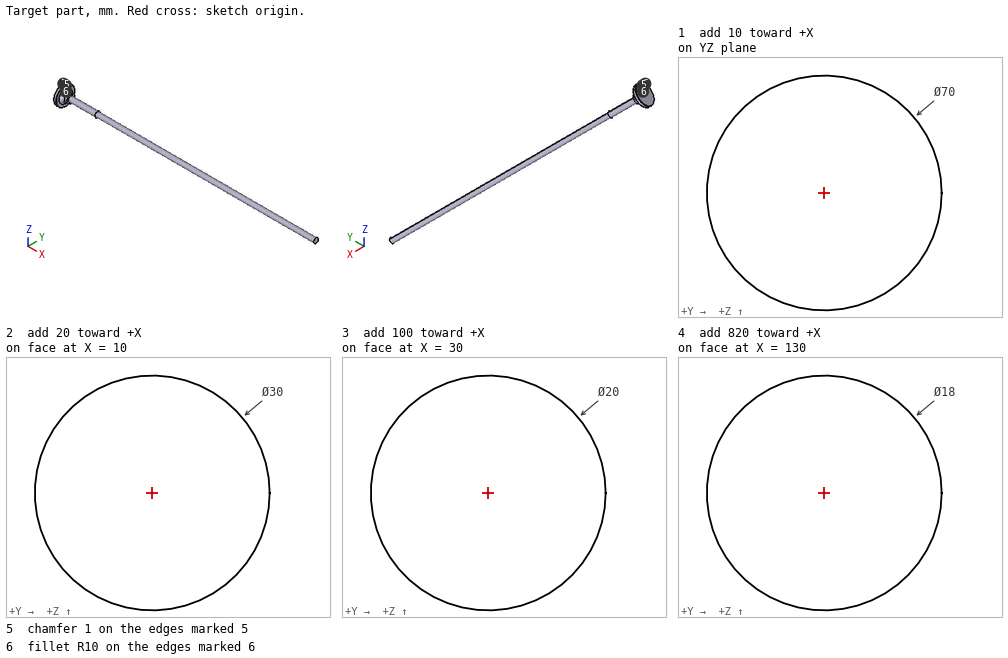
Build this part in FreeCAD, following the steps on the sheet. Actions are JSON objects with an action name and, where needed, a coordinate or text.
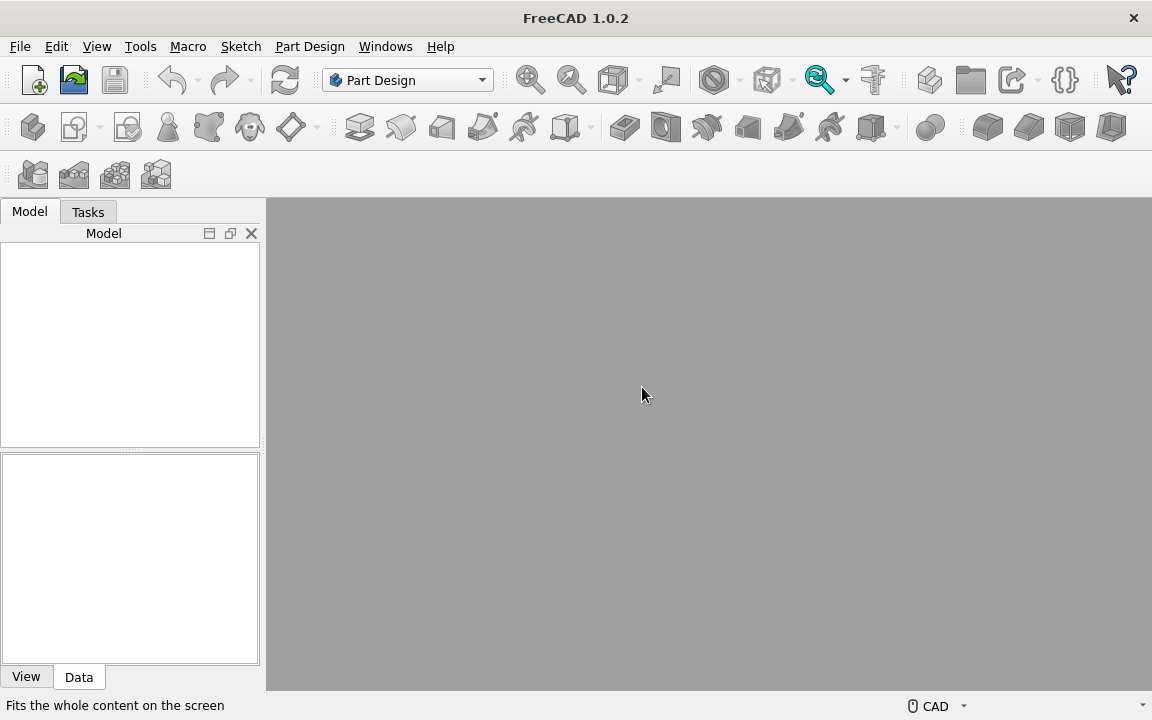
{"action": "left_click", "coordinate": [33, 80]}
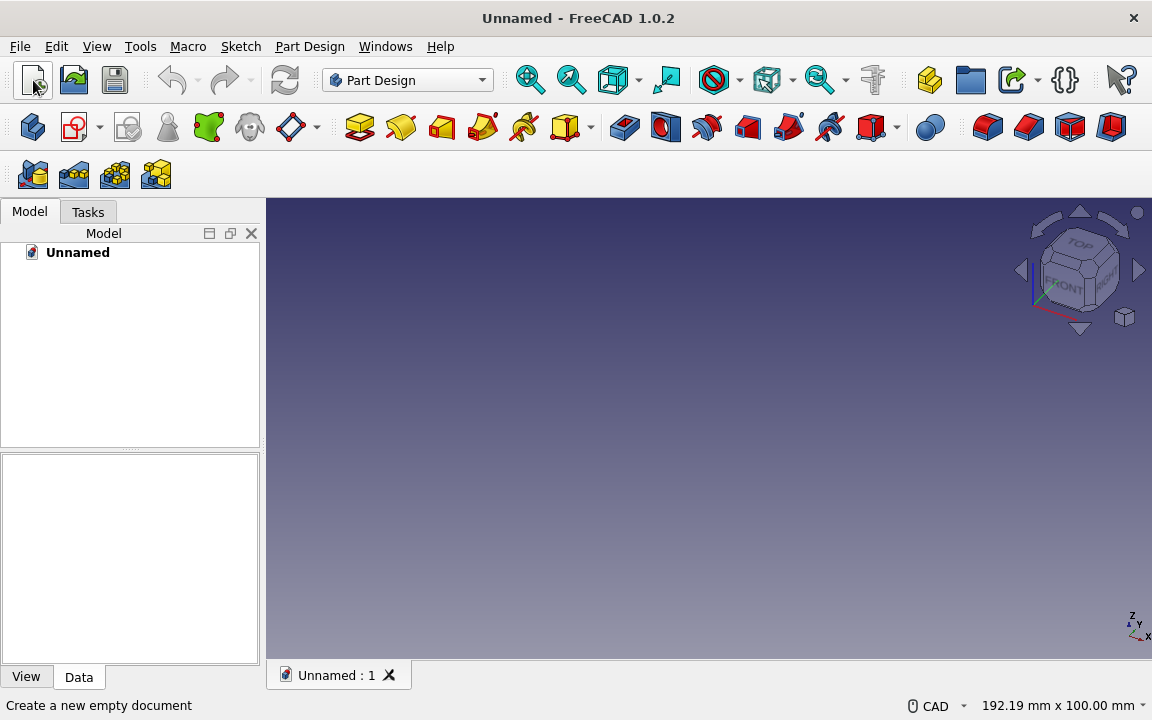
{"action": "left_click", "coordinate": [74, 128]}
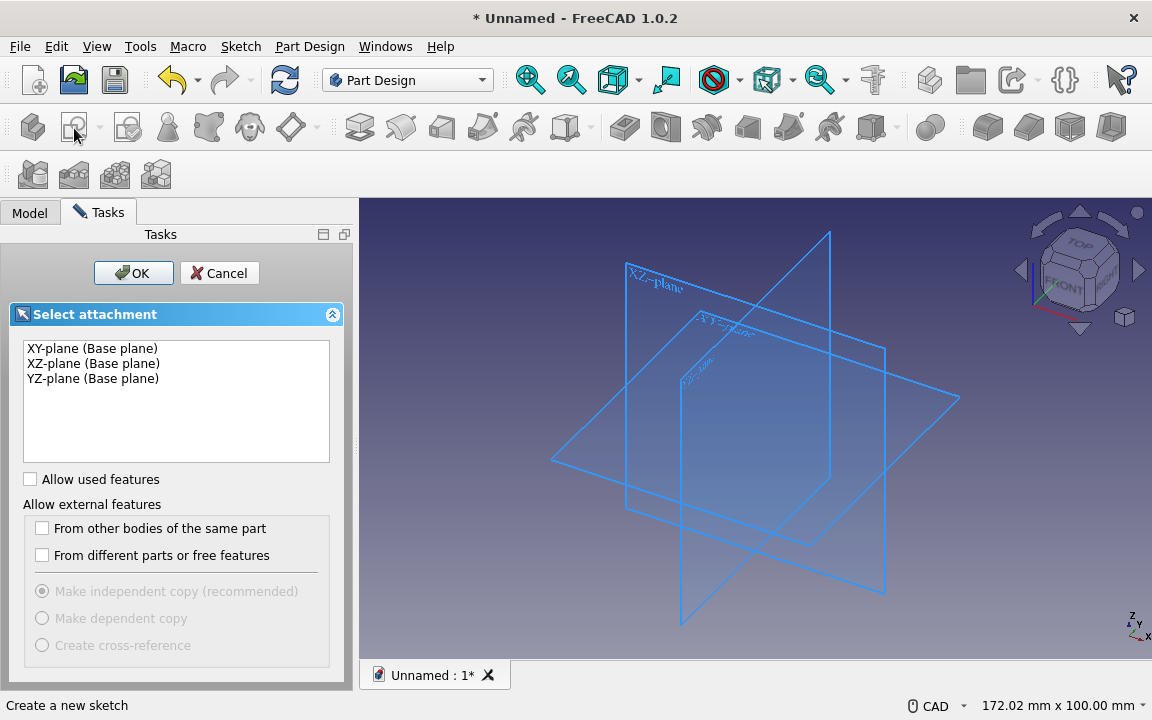
{"action": "left_click", "coordinate": [84, 378]}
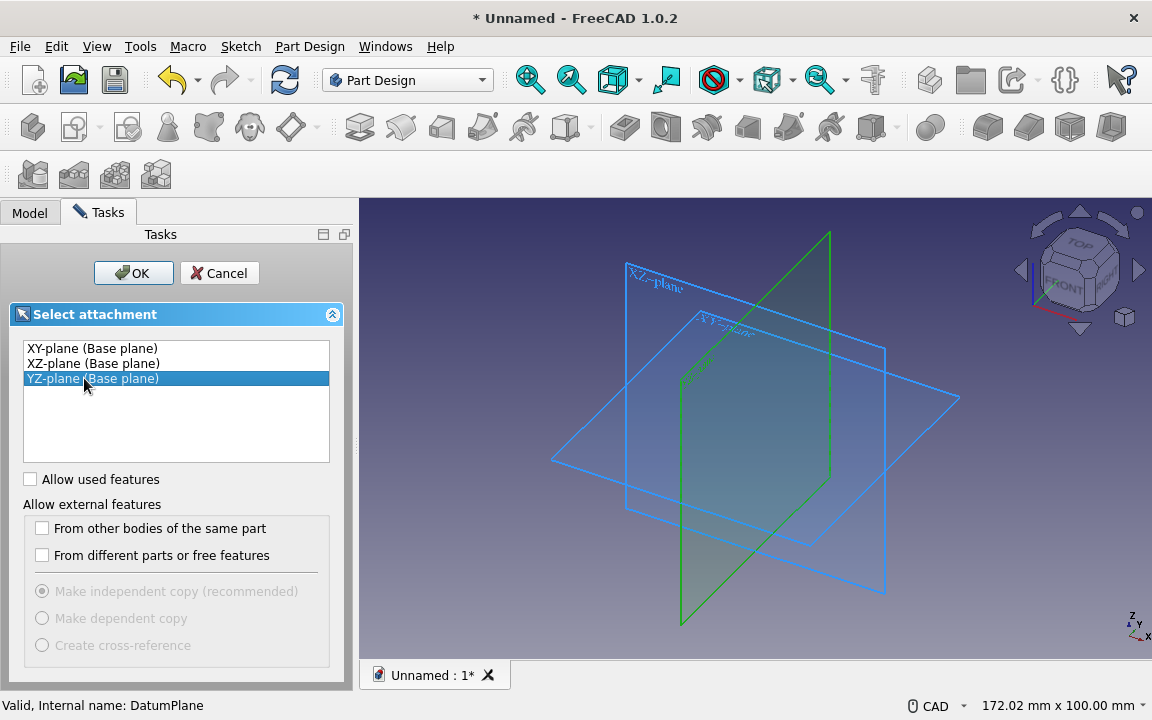
{"action": "left_click", "coordinate": [134, 273]}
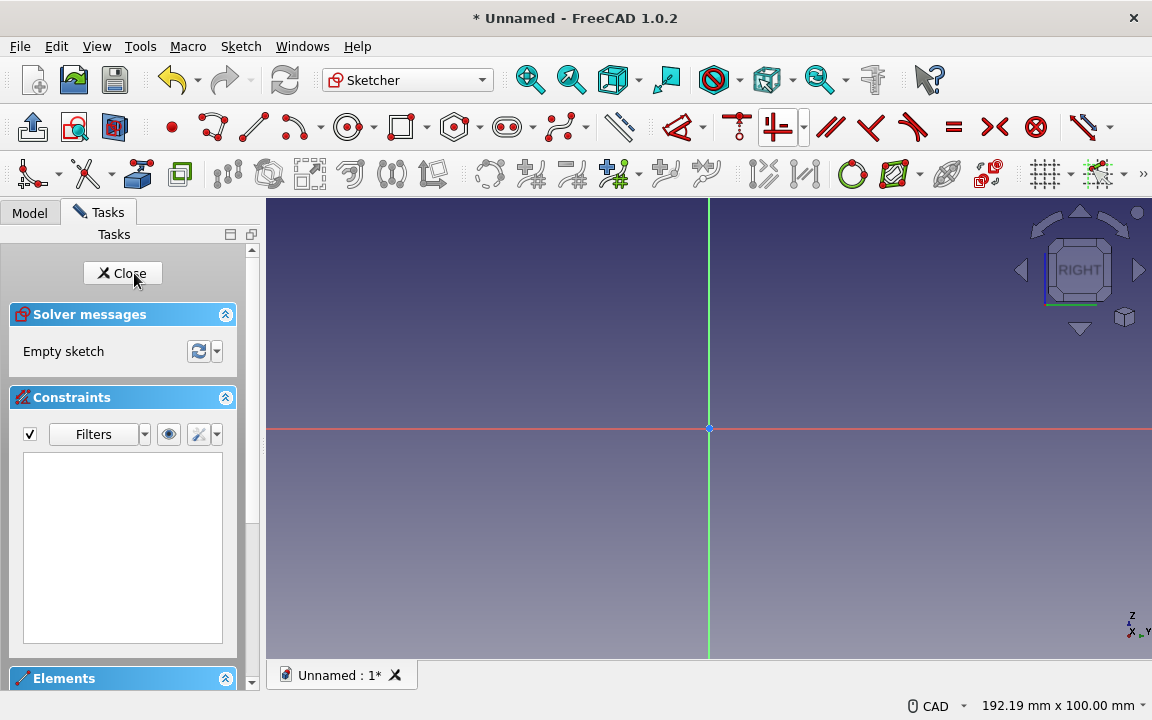
{"action": "left_click", "coordinate": [348, 128]}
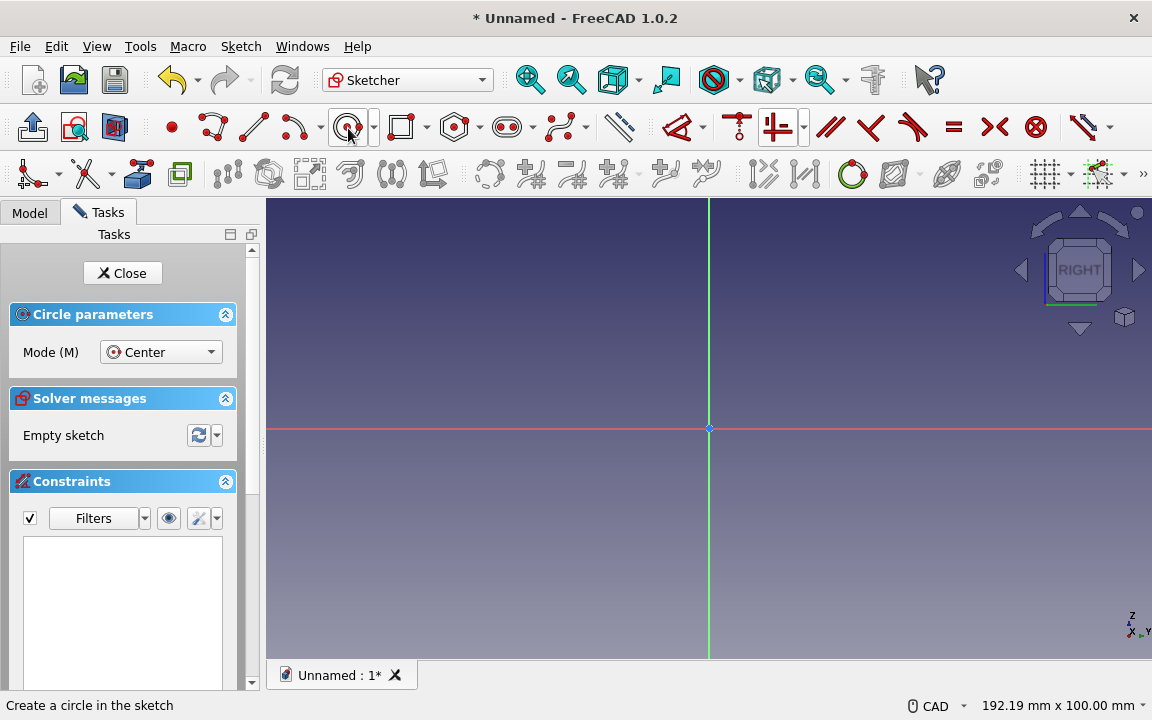
{"action": "left_click", "coordinate": [709, 428]}
{"action": "left_click", "coordinate": [823, 314]}
{"action": "key", "text": "Escape"}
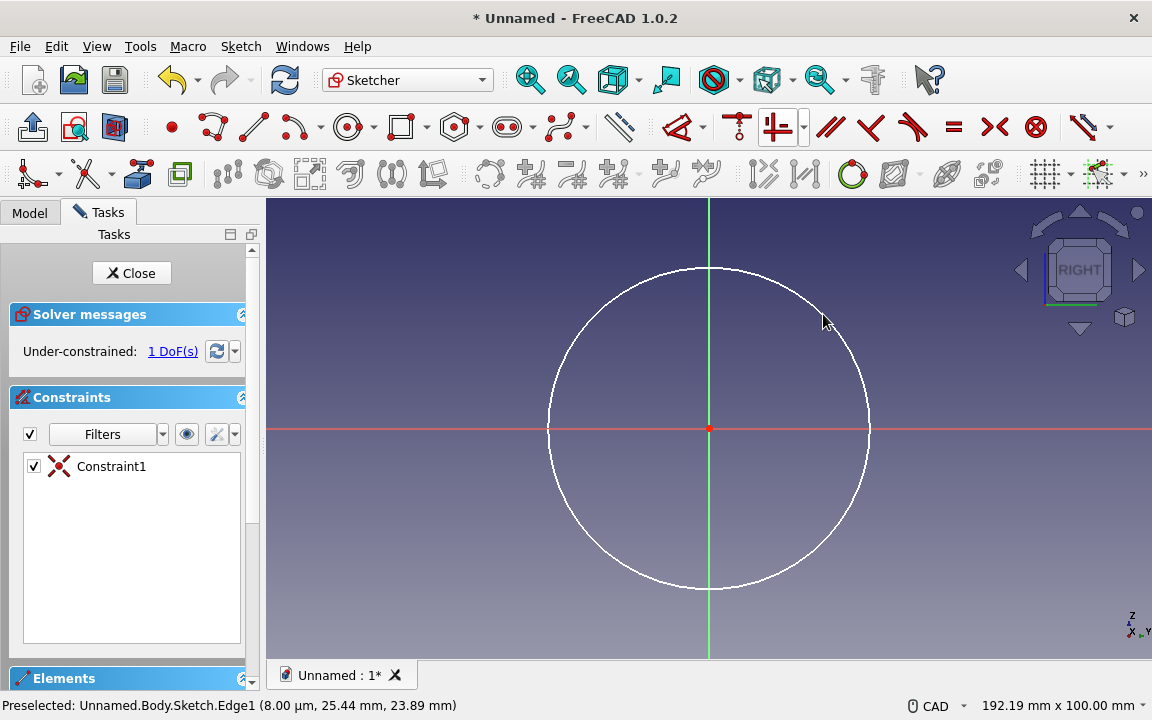
{"action": "key", "text": "d"}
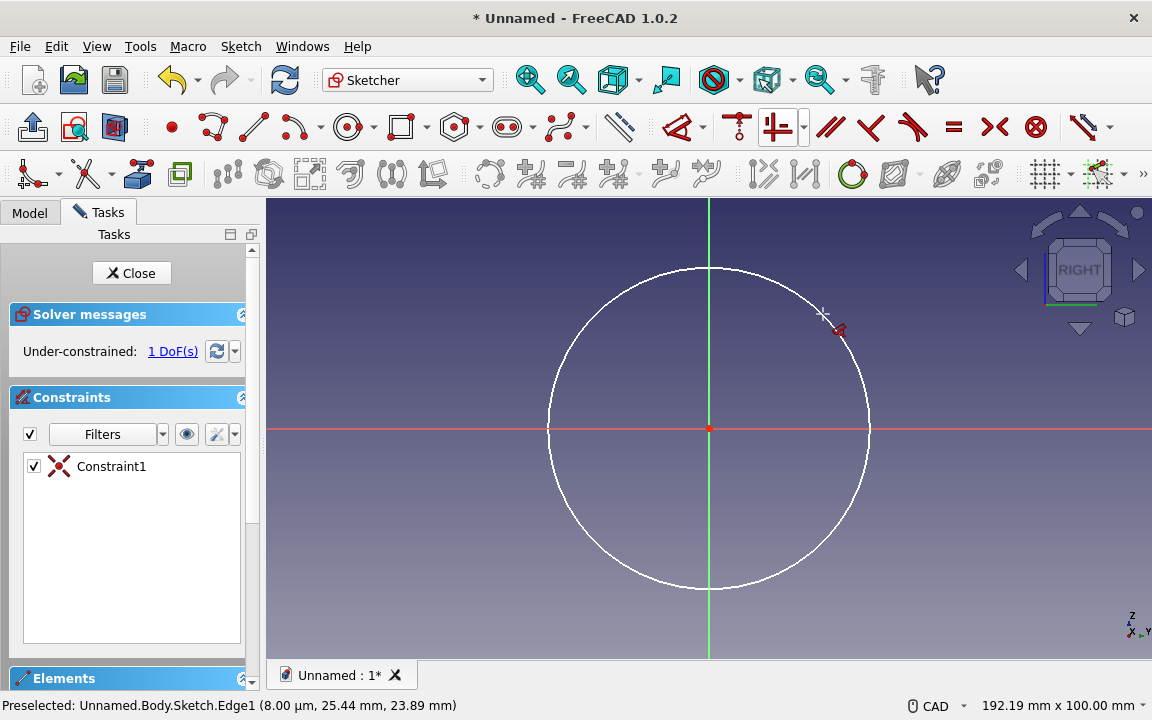
{"action": "left_click", "coordinate": [822, 314]}
{"action": "left_click", "coordinate": [844, 291]}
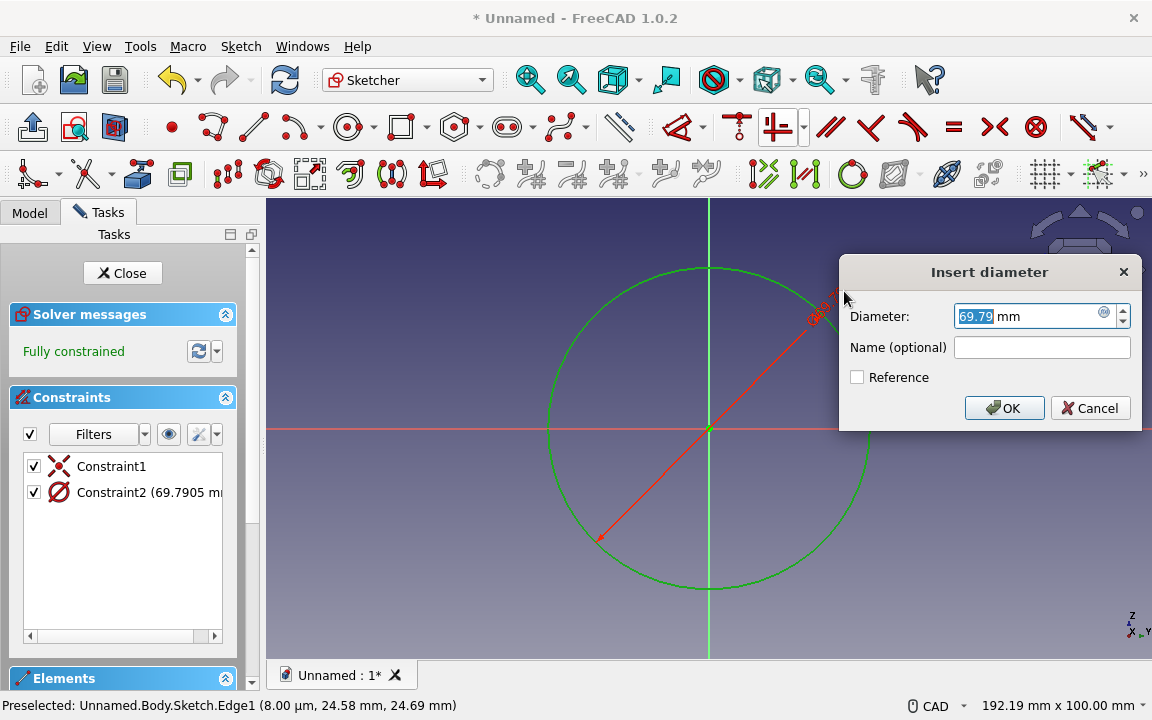
{"action": "type", "text": "70"}
{"action": "key", "text": "Return"}
{"action": "key", "text": "Escape"}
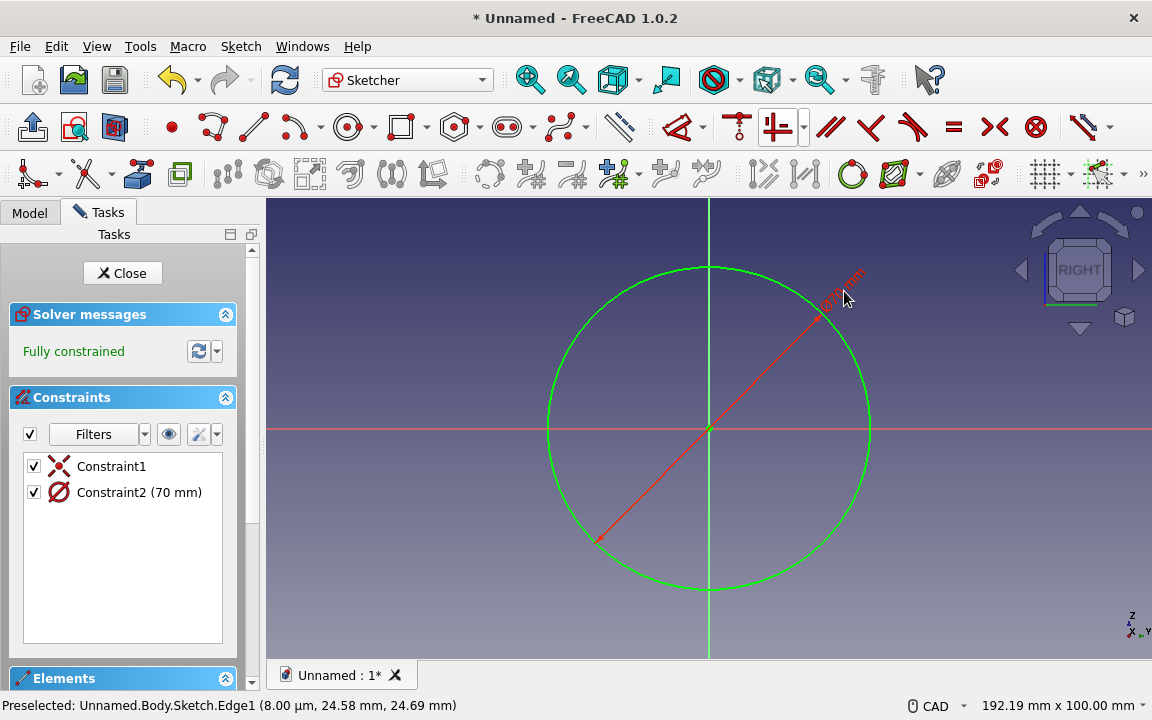
{"action": "left_click", "coordinate": [123, 273]}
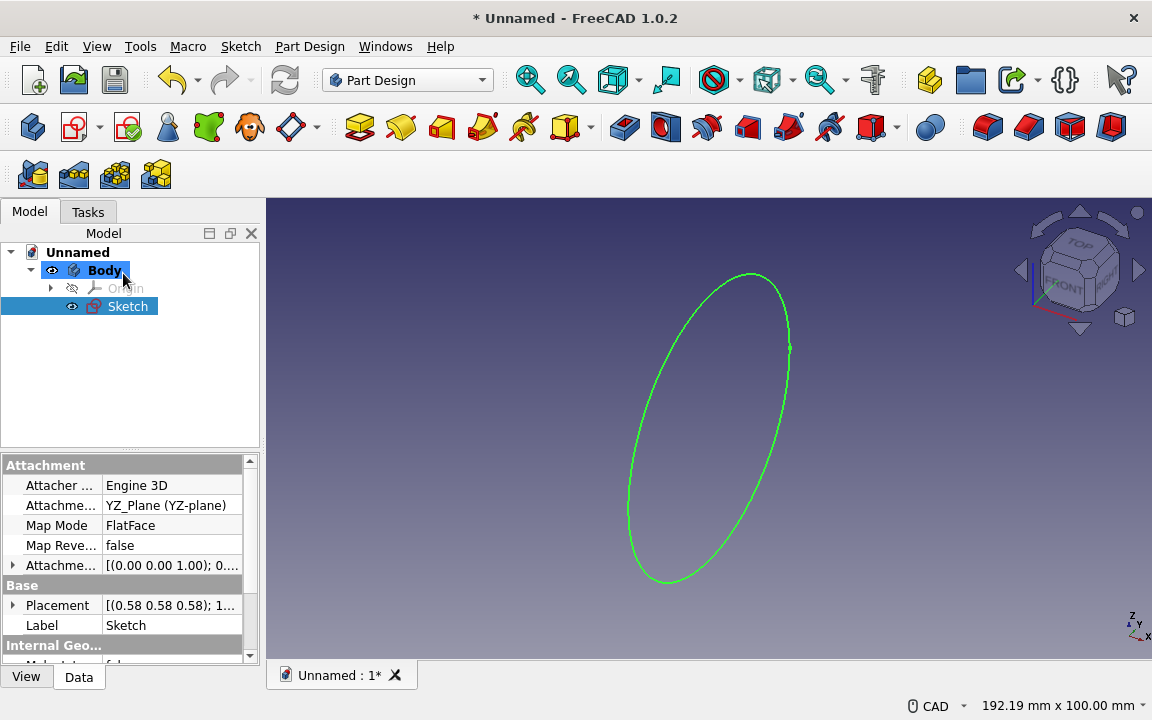
{"action": "left_click", "coordinate": [360, 128]}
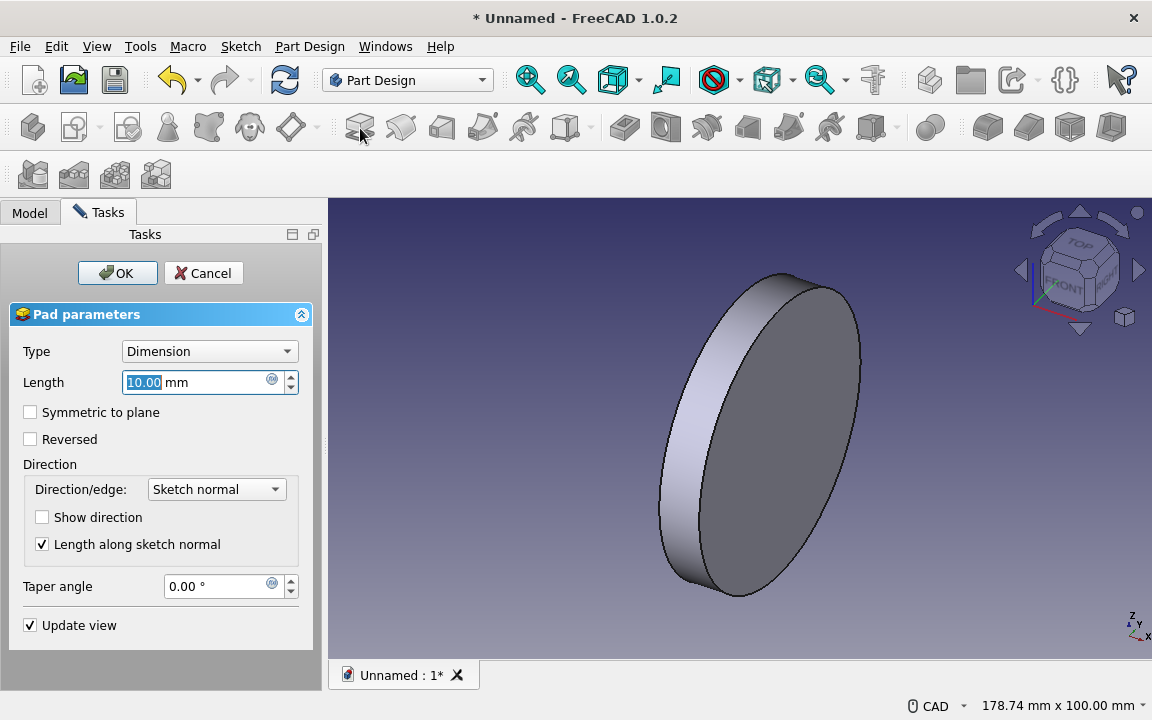
{"action": "type", "text": "10"}
{"action": "key", "text": "Tab"}